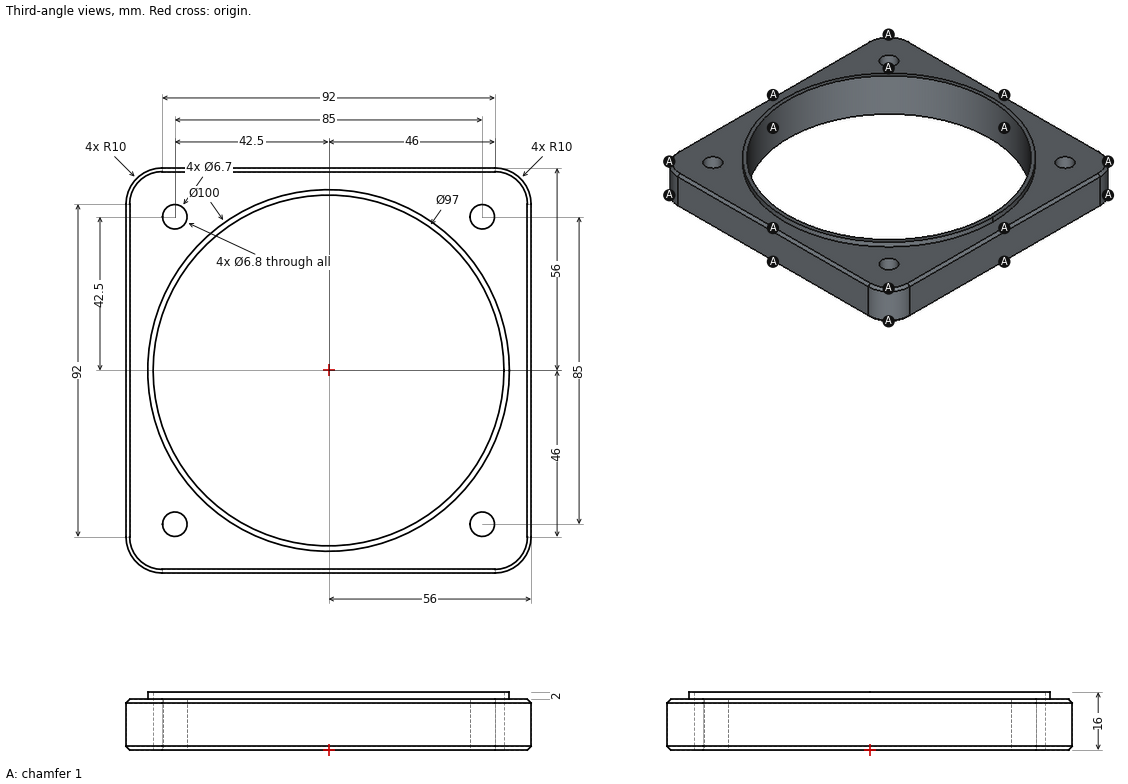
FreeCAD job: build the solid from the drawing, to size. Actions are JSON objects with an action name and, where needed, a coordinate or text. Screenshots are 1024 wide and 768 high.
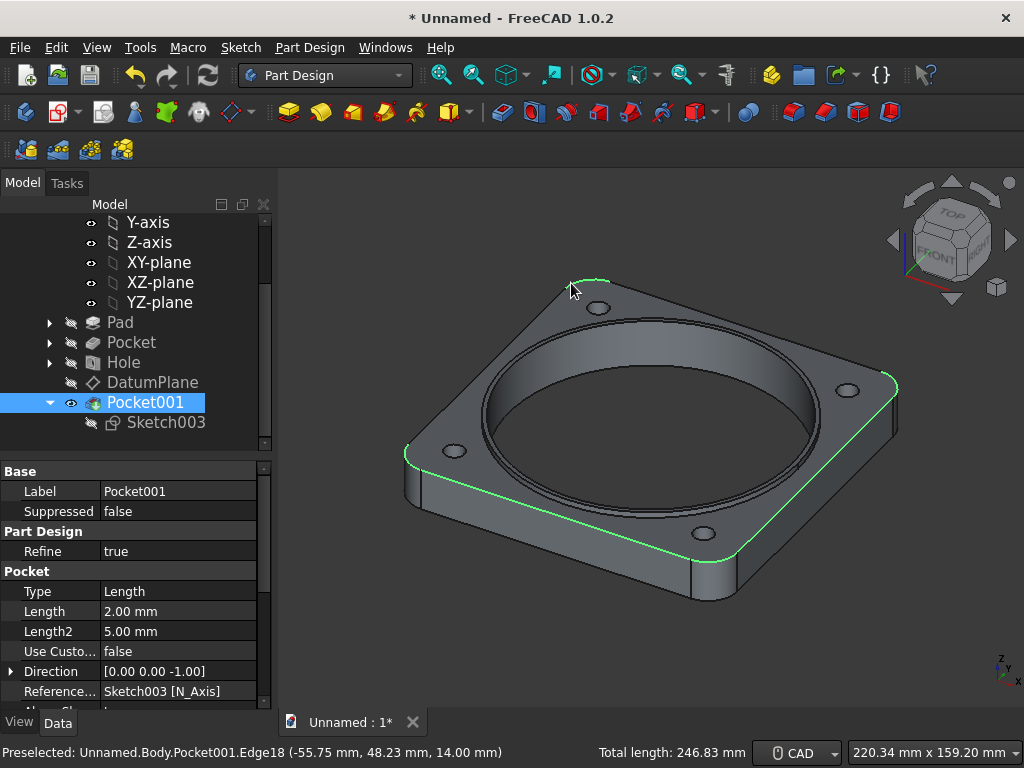
{"action": "key", "text": "0"}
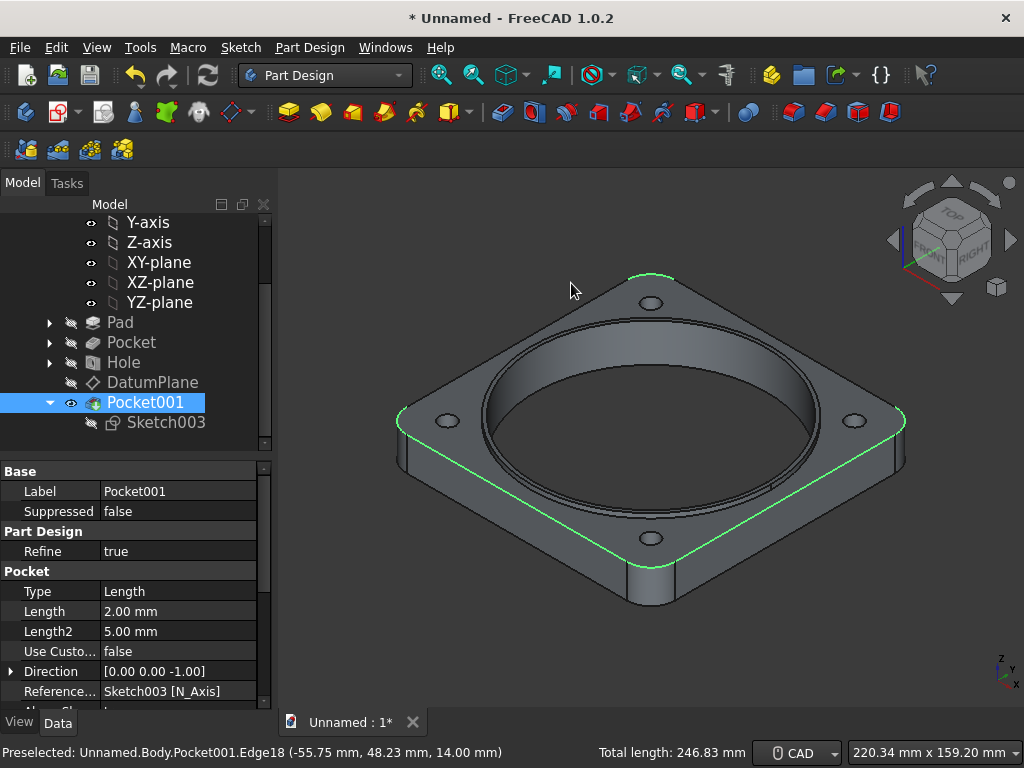
{"action": "key", "text": "2"}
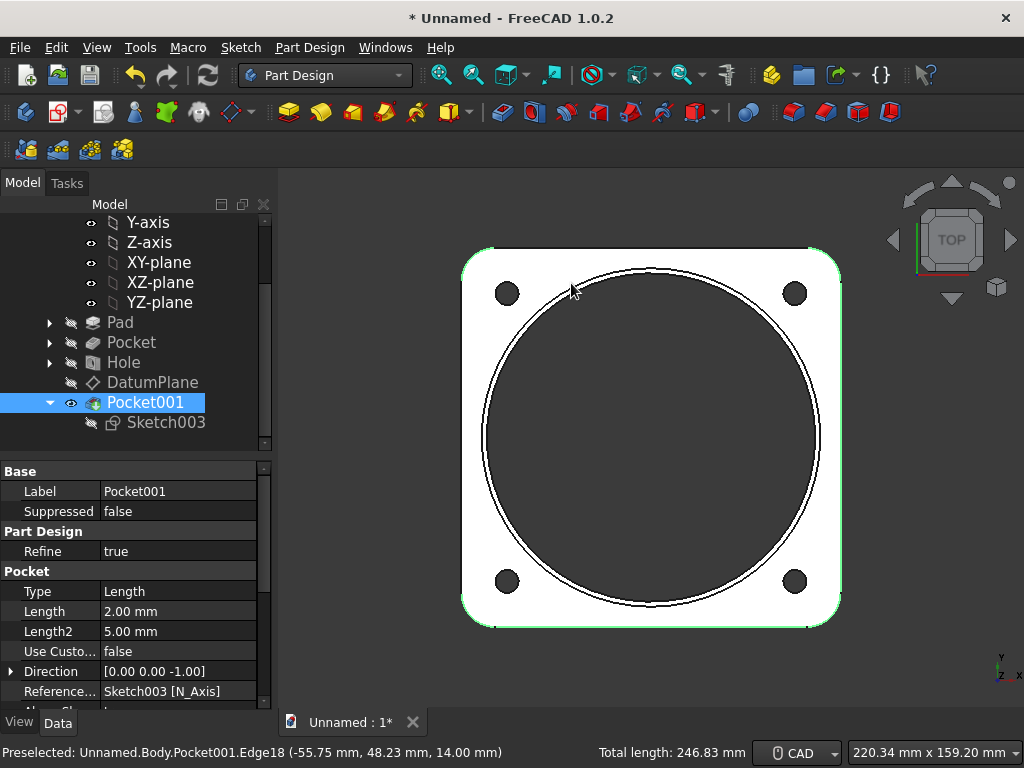
{"action": "left_click", "coordinate": [461, 437], "text": "ctrl"}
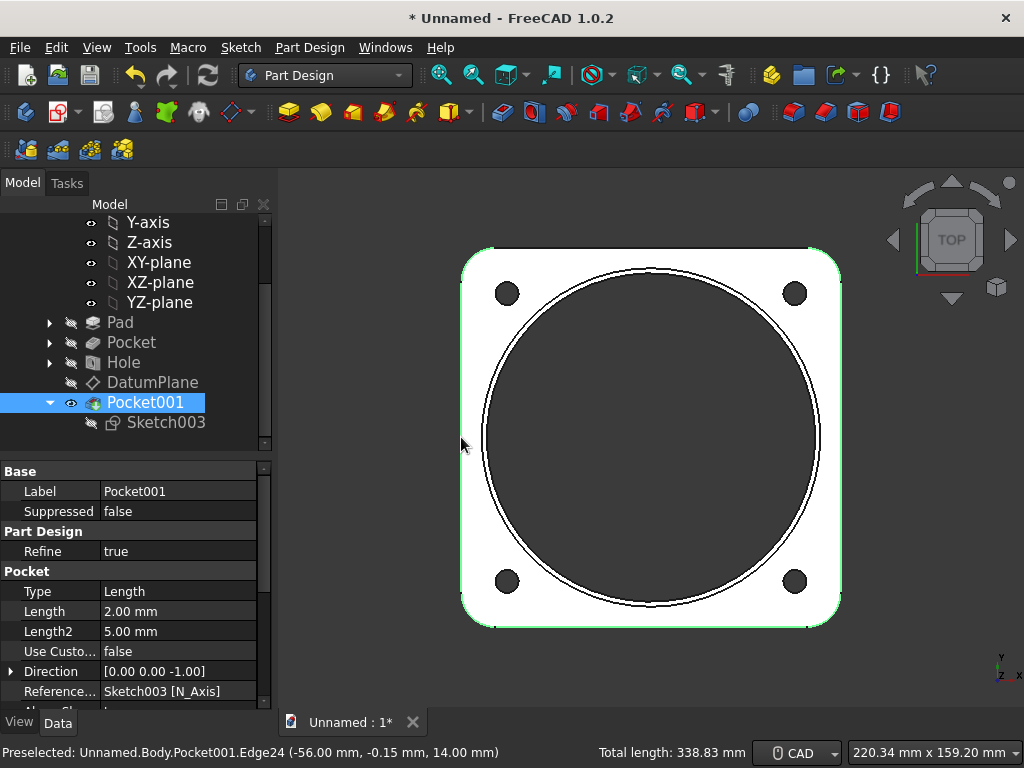
{"action": "left_click", "coordinate": [651, 247], "text": "ctrl"}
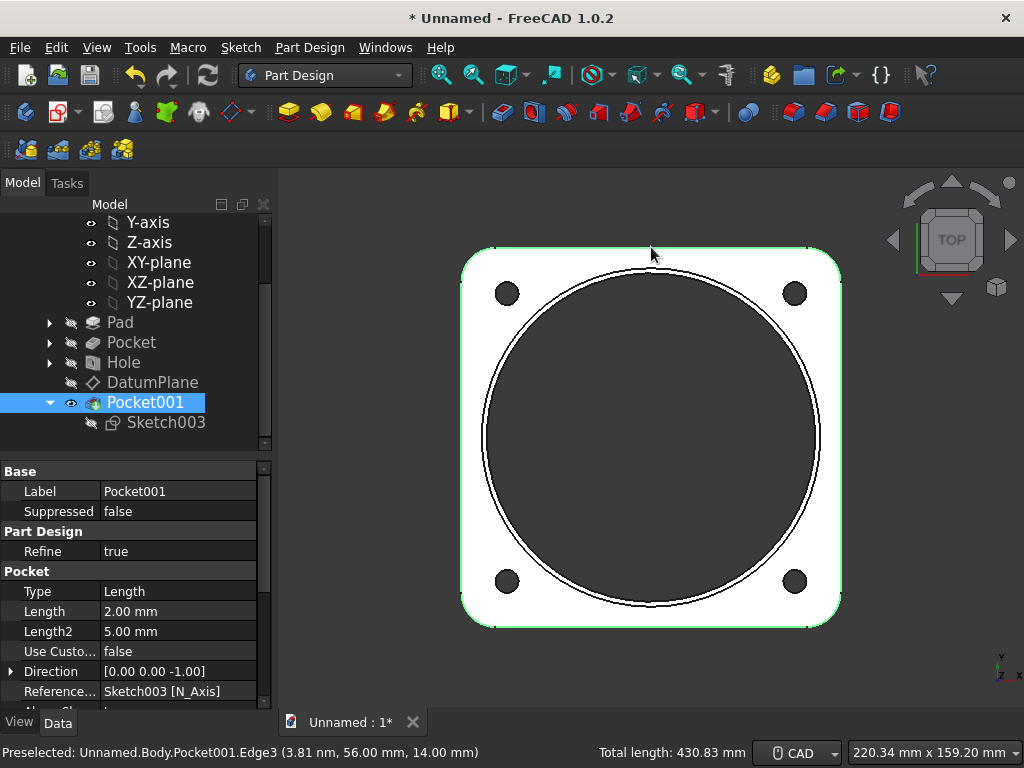
{"action": "key", "text": "1"}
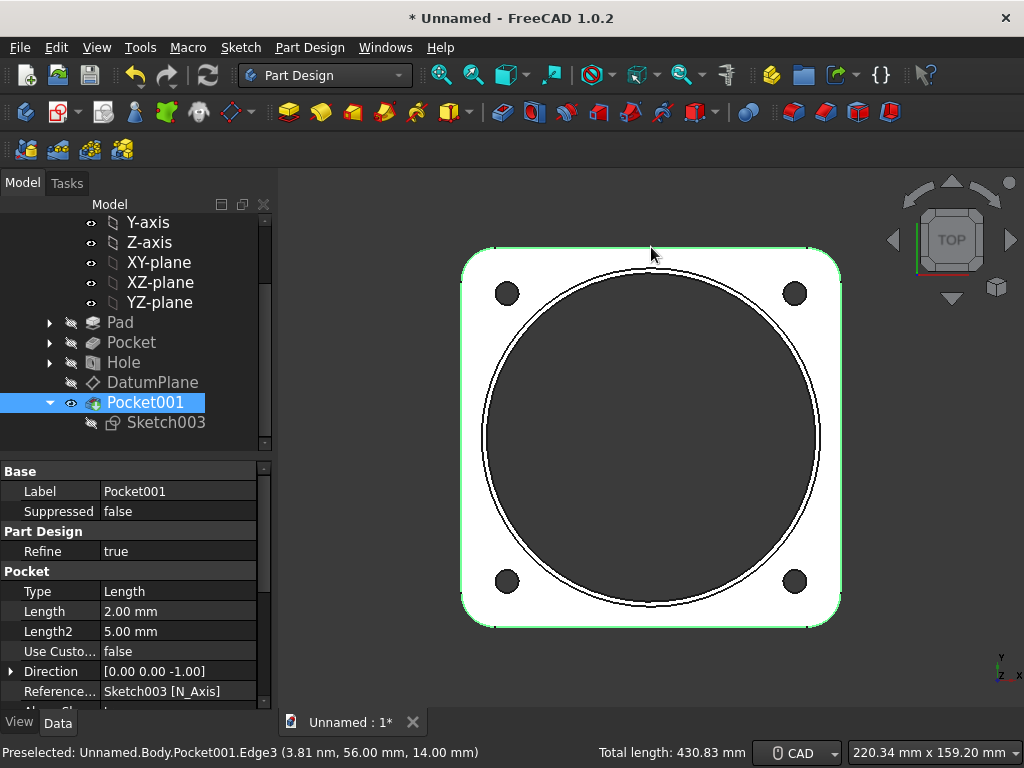
{"action": "left_click", "coordinate": [831, 464], "text": "ctrl"}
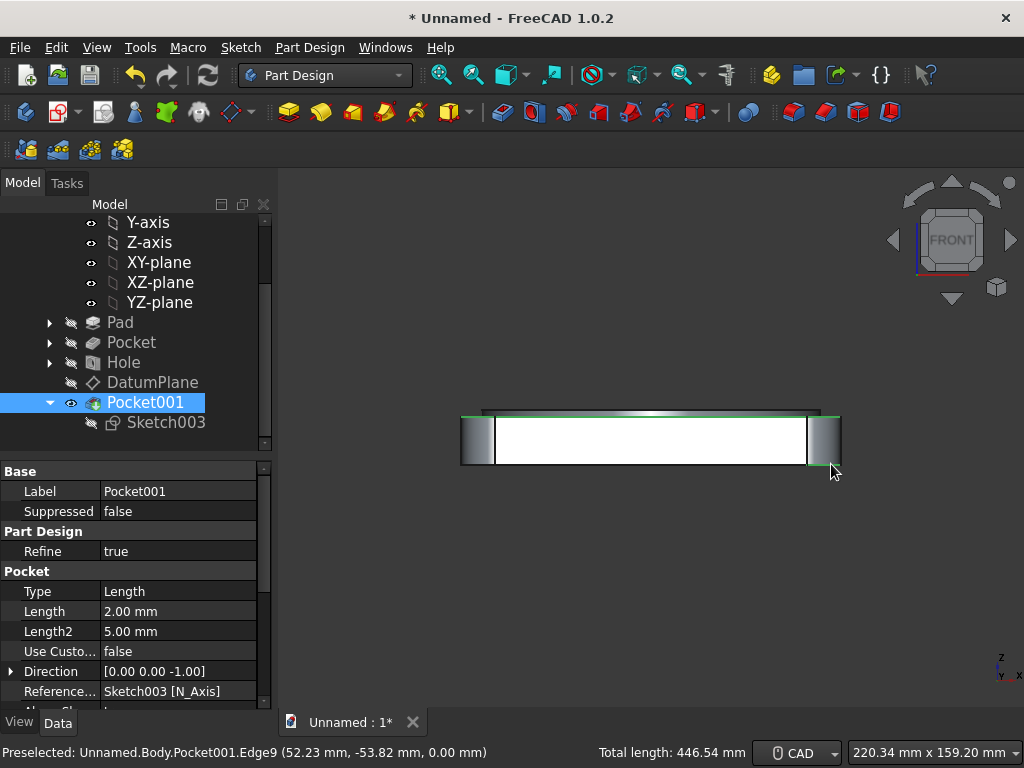
{"action": "left_click", "coordinate": [651, 464], "text": "ctrl"}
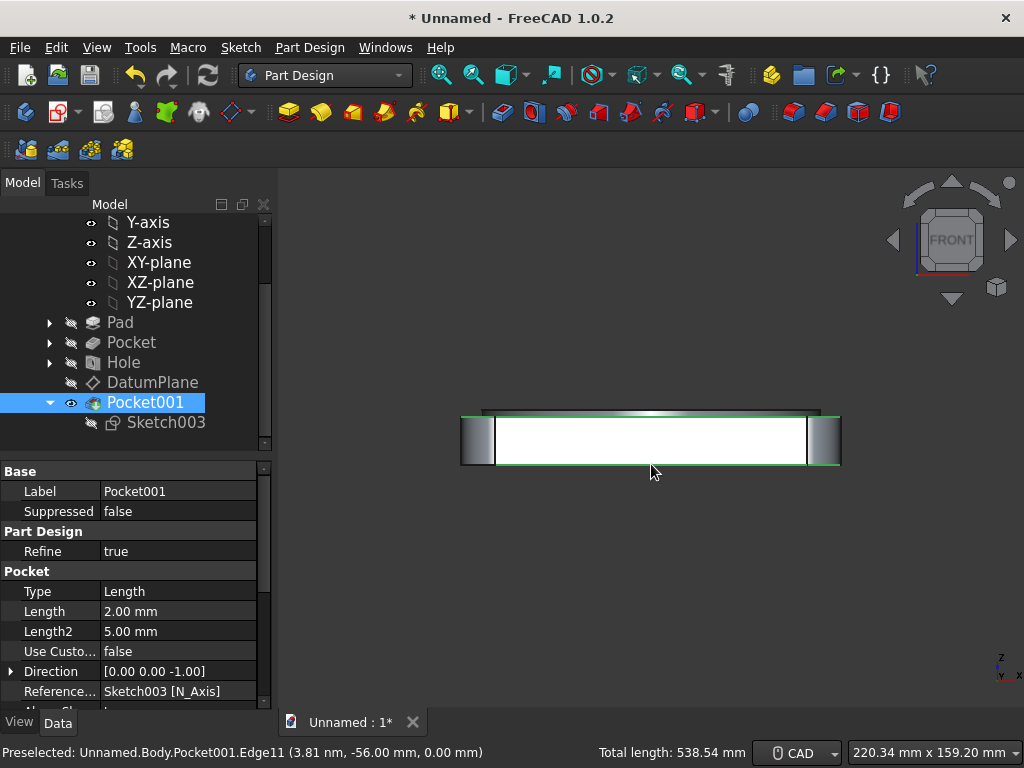
{"action": "left_click", "coordinate": [471, 464], "text": "ctrl"}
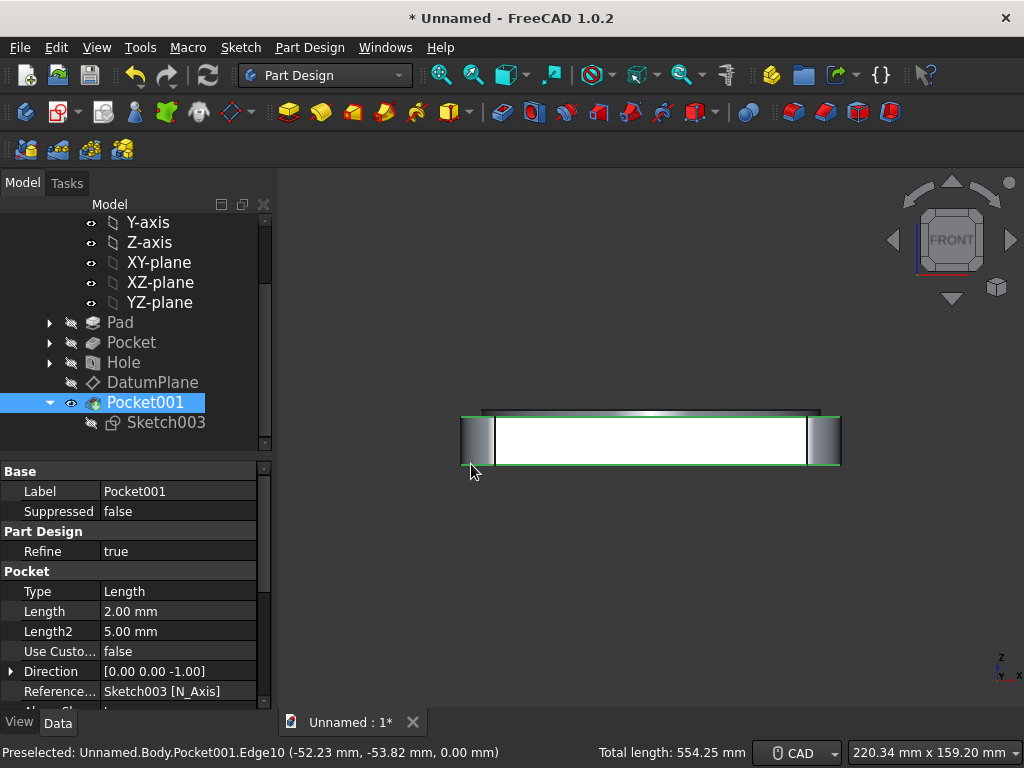
{"action": "key", "text": "3"}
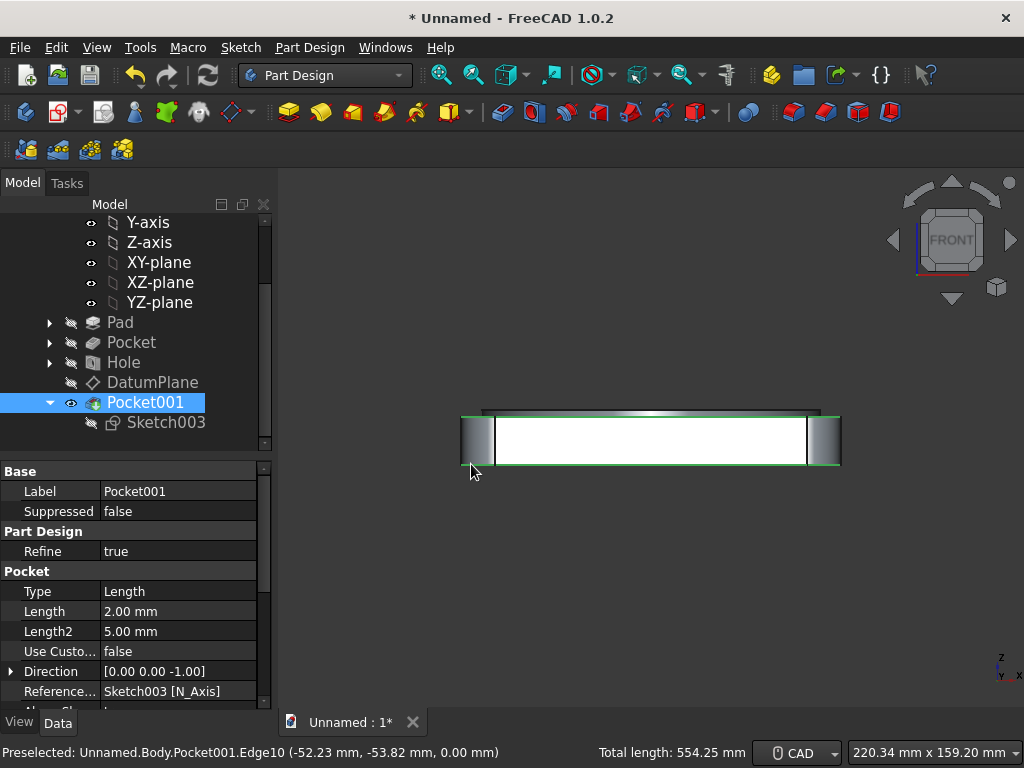
{"action": "left_click", "coordinate": [651, 464], "text": "ctrl"}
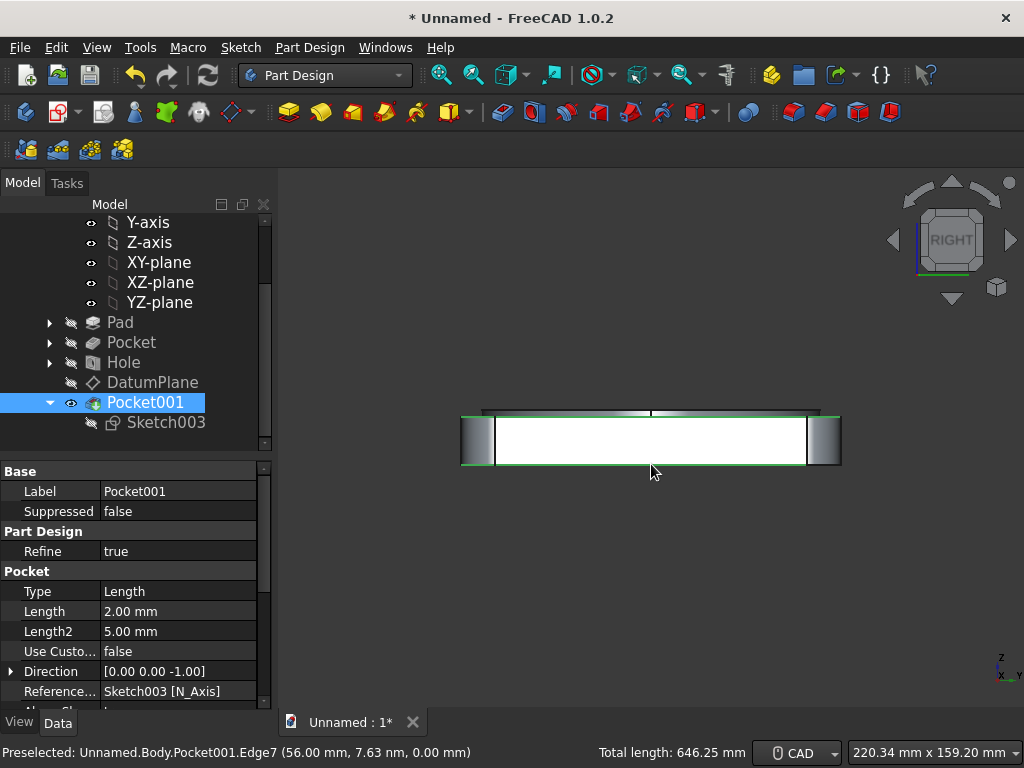
{"action": "left_click", "coordinate": [831, 464], "text": "ctrl"}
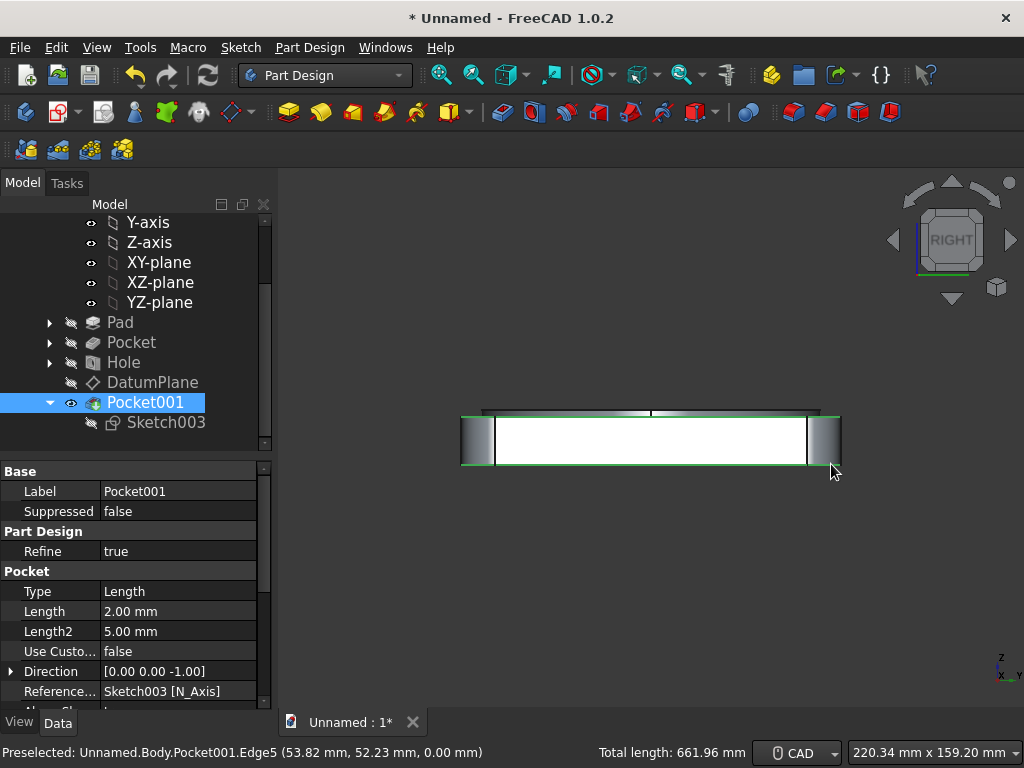
{"action": "key", "text": "5"}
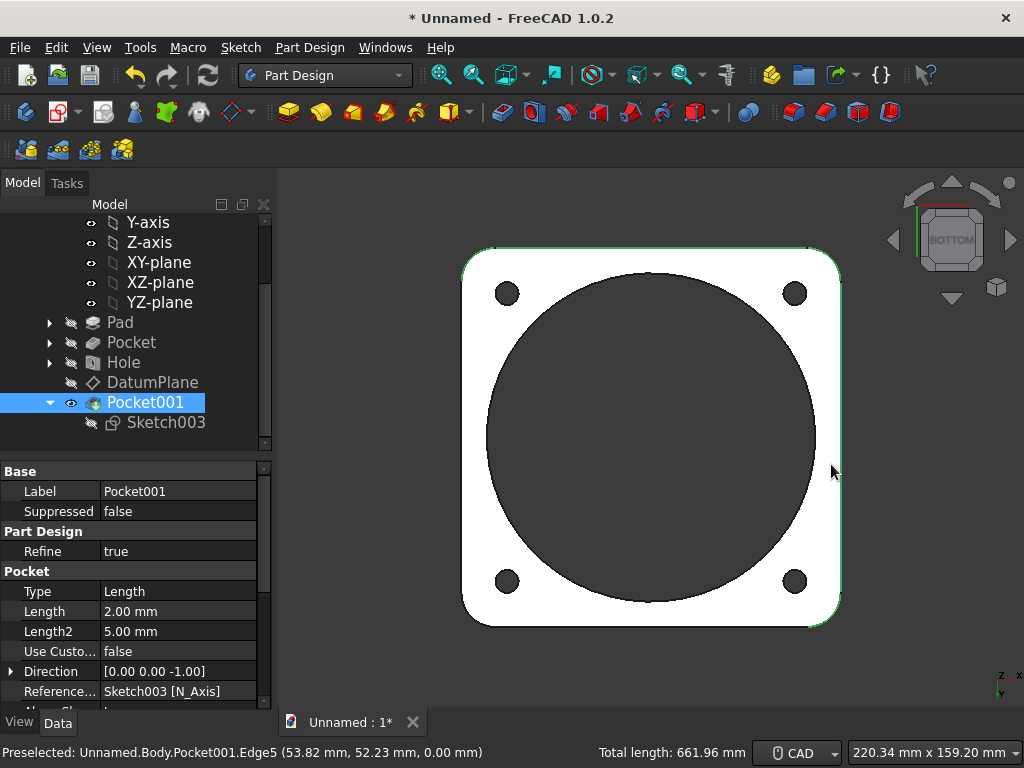
{"action": "left_click", "coordinate": [461, 436], "text": "ctrl"}